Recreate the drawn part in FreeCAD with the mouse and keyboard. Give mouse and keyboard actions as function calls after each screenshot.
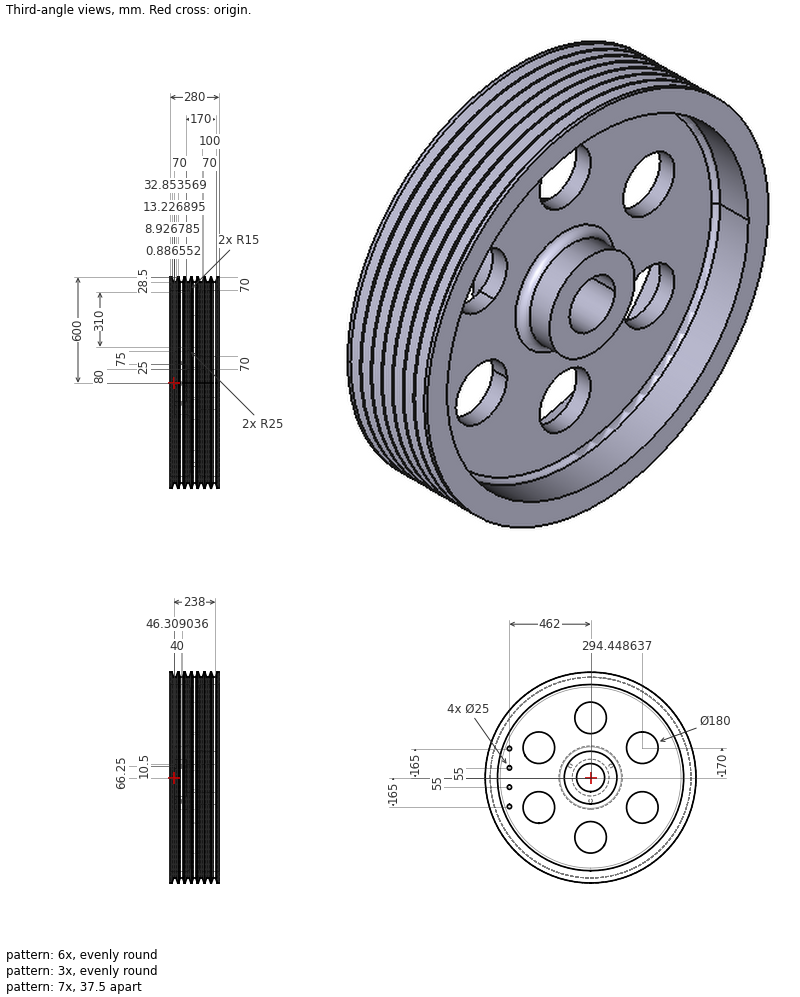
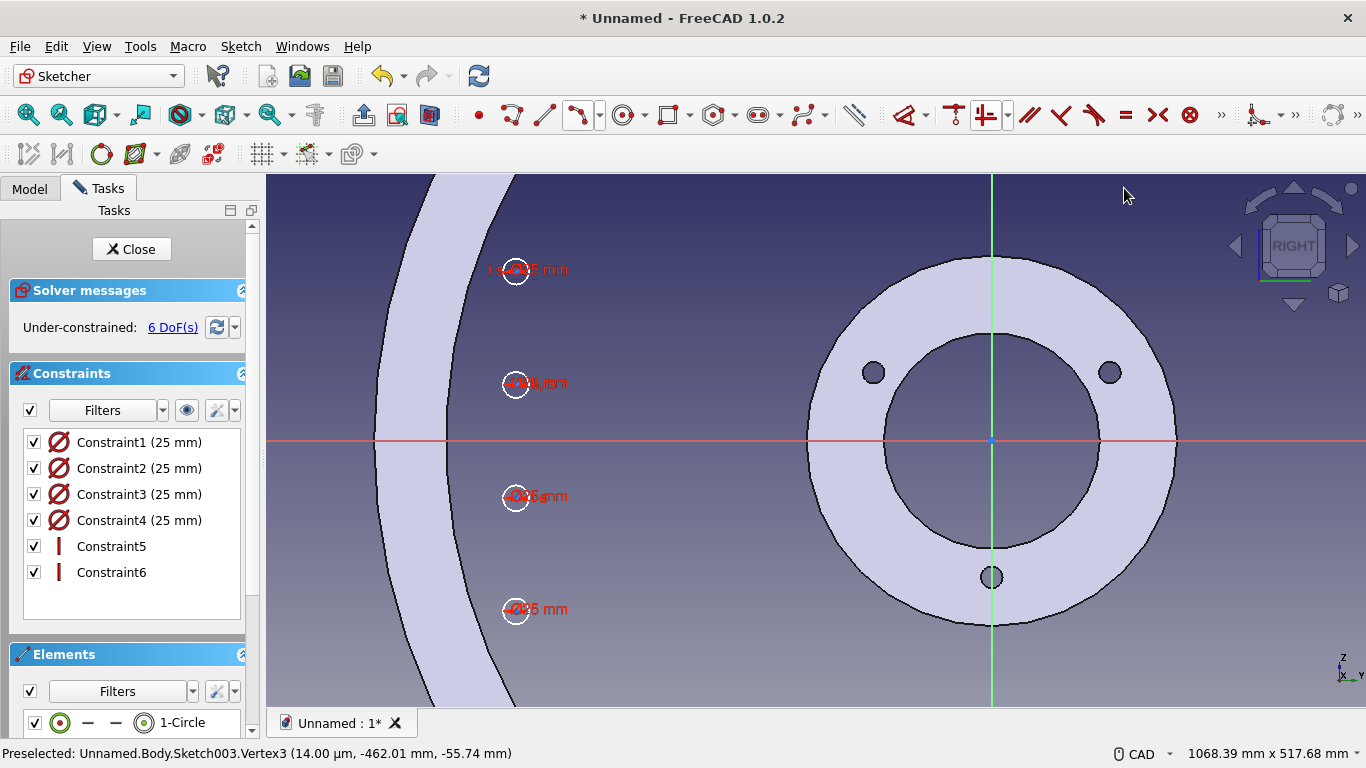
click(516, 498)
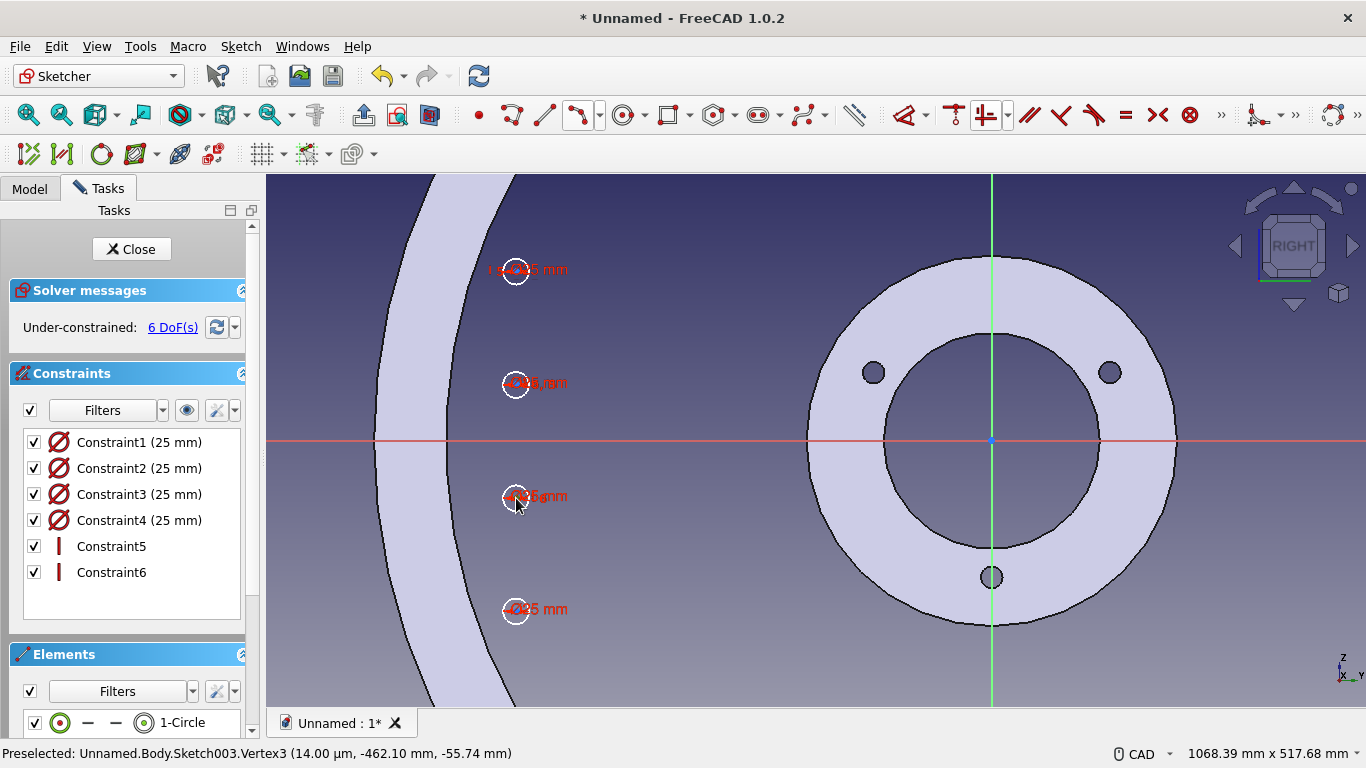
click(516, 611)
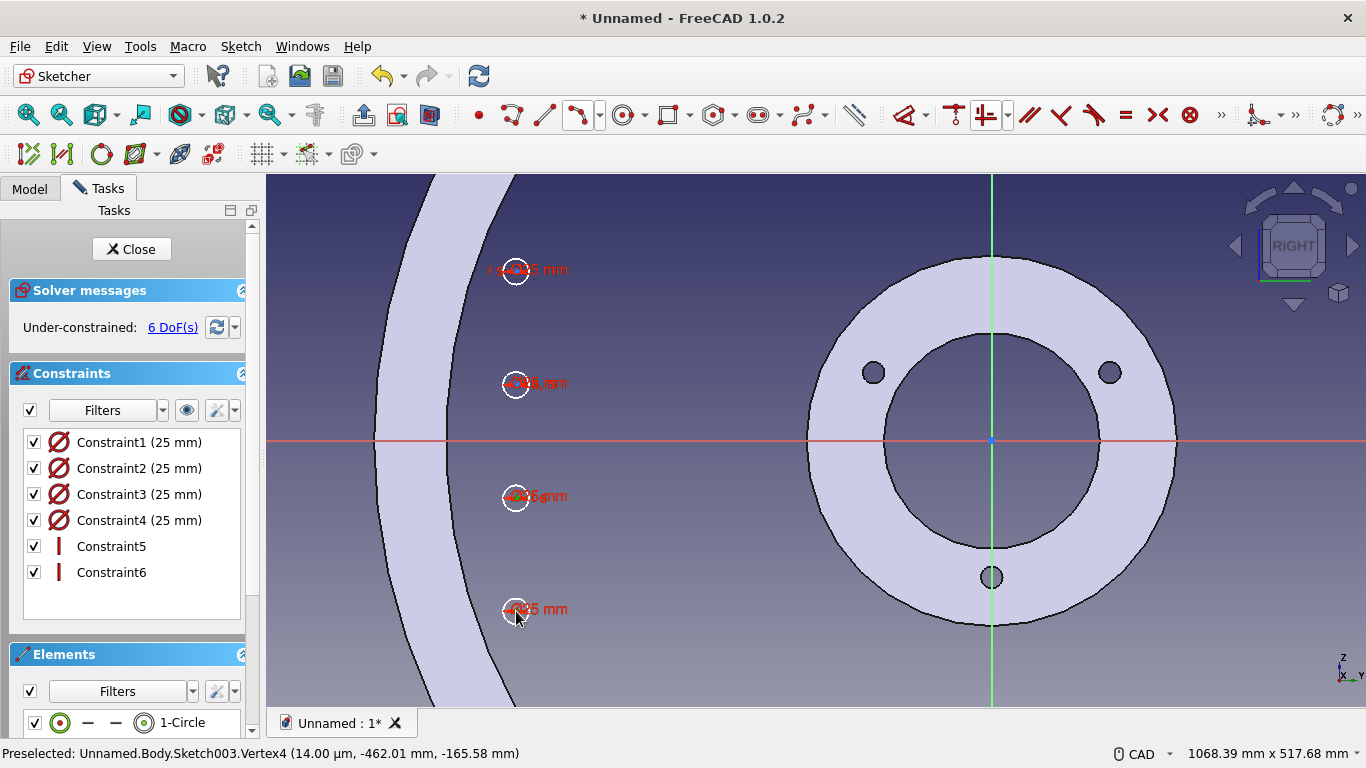
click(1008, 116)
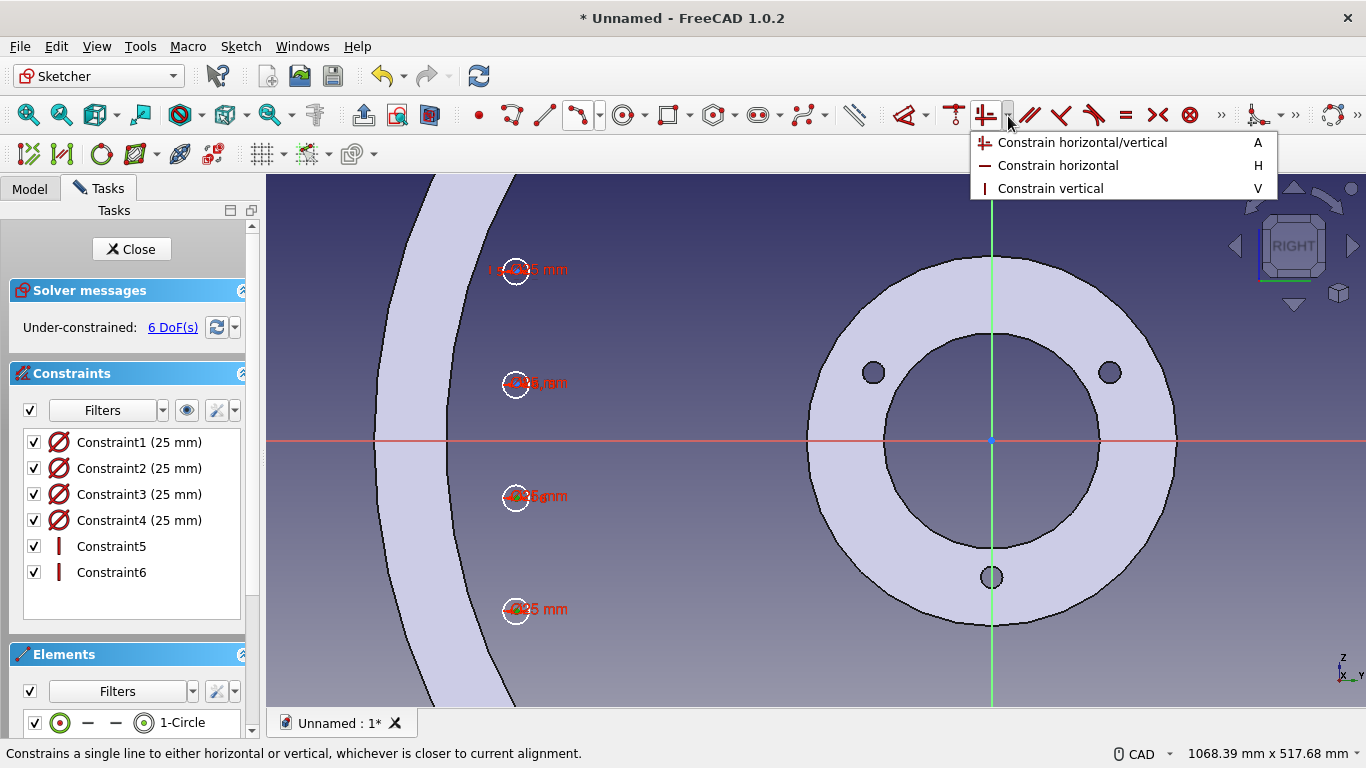
click(1124, 188)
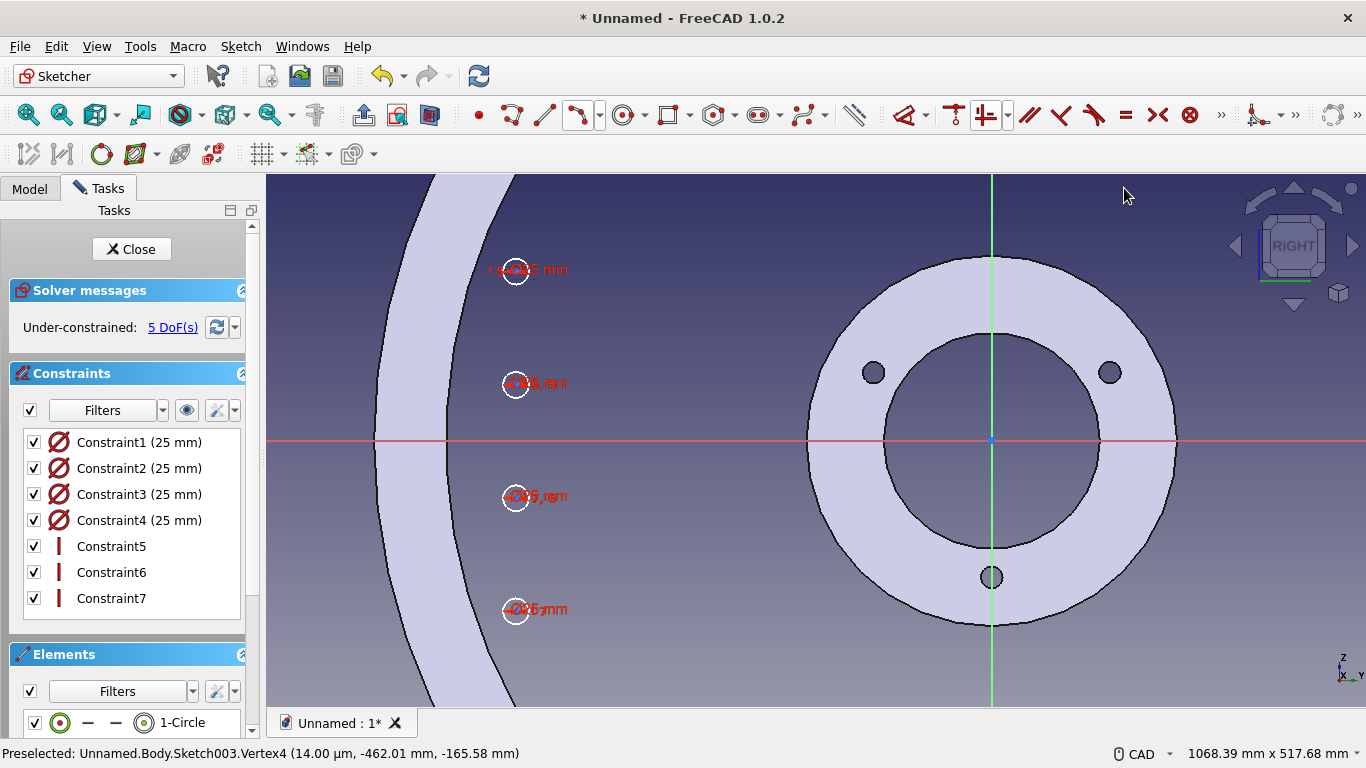
click(904, 116)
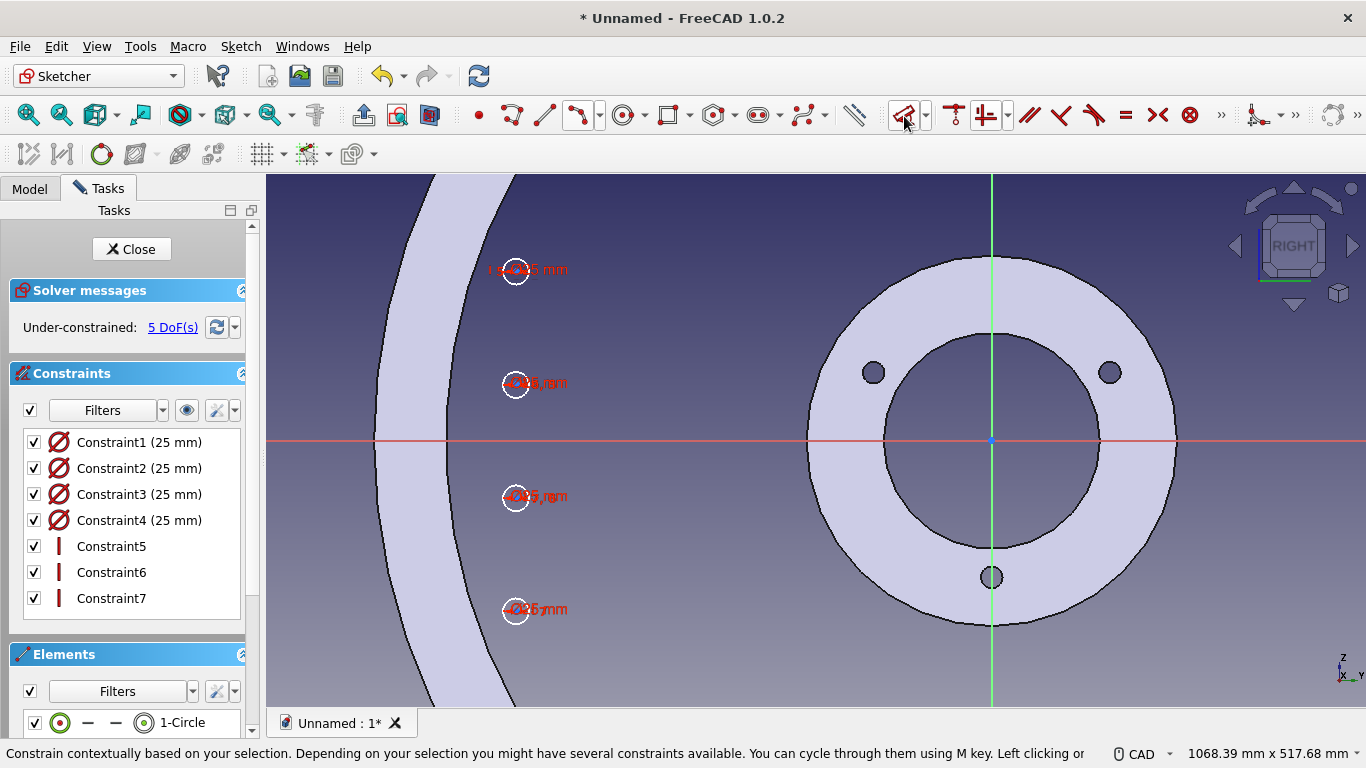
click(516, 385)
click(1026, 413)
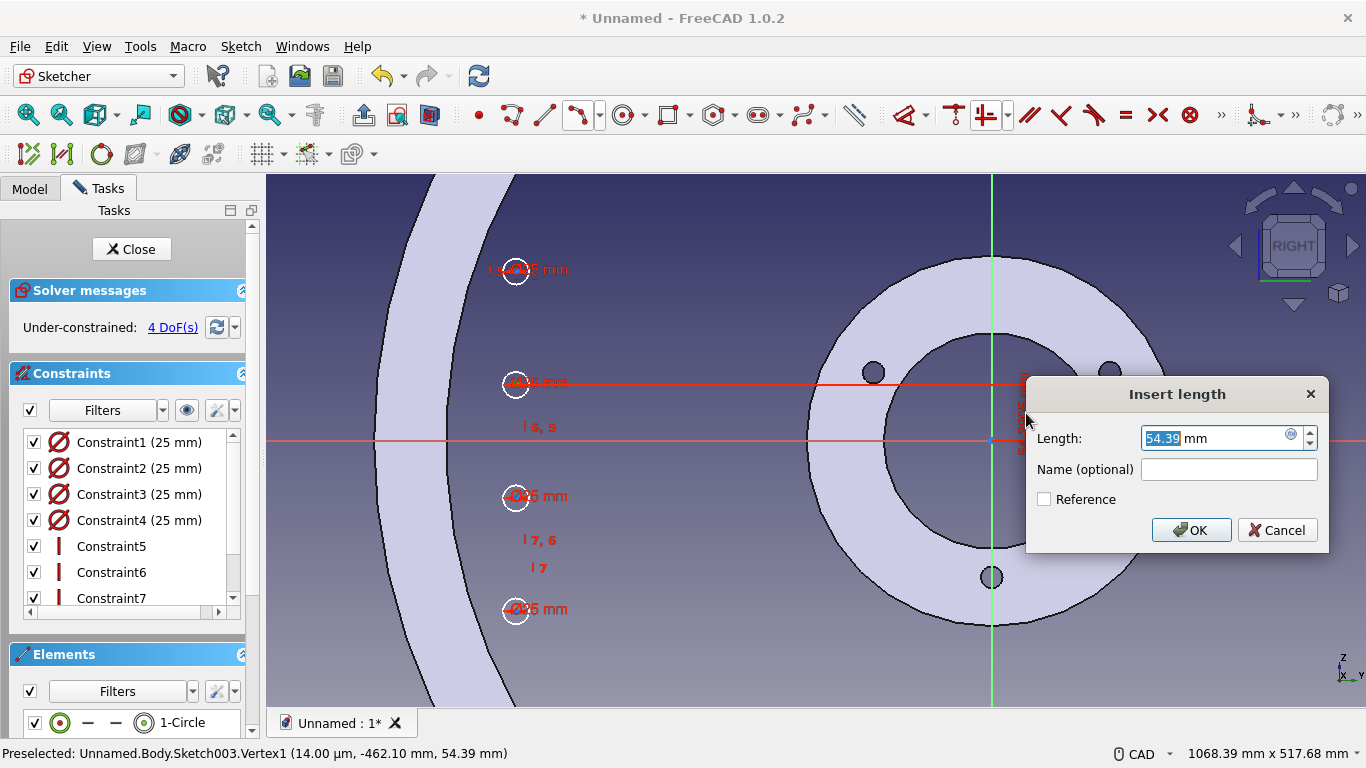
text(55)
key(Return)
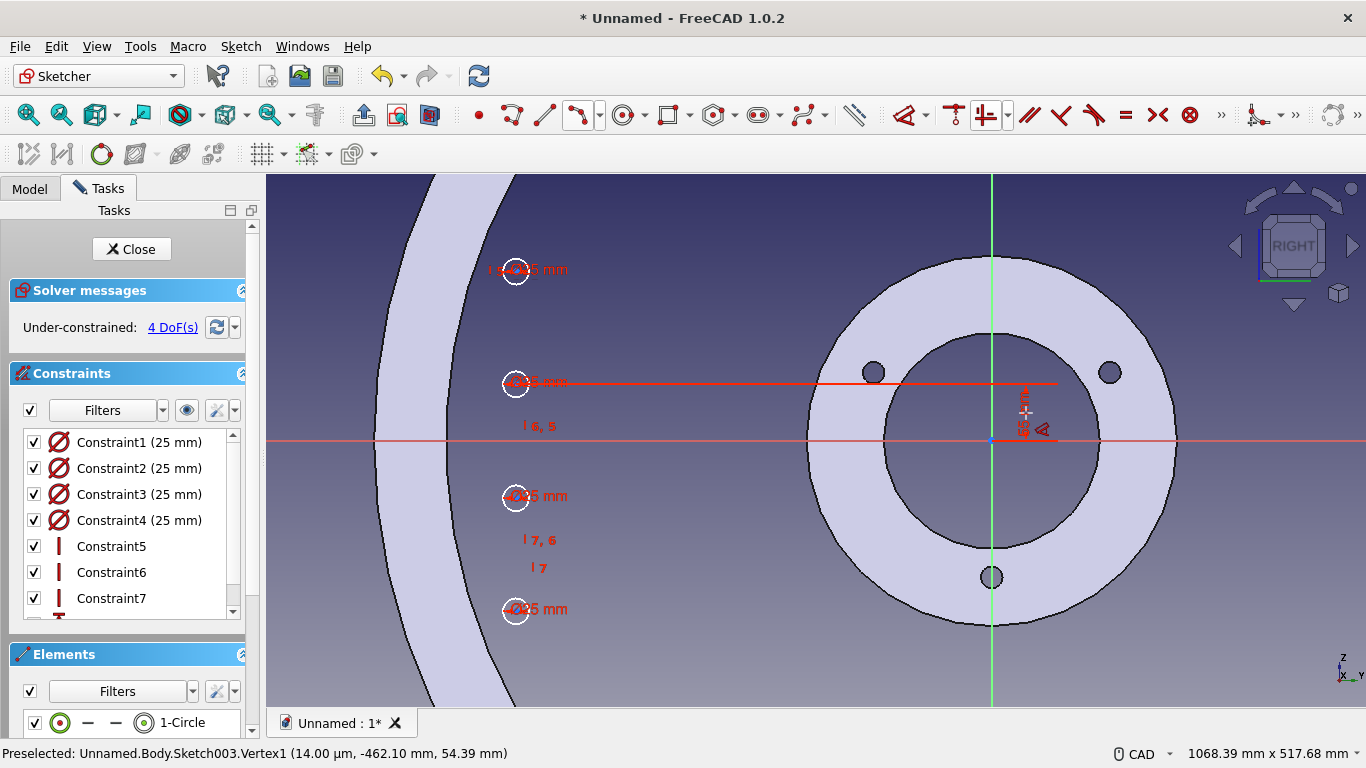
click(516, 498)
click(1026, 470)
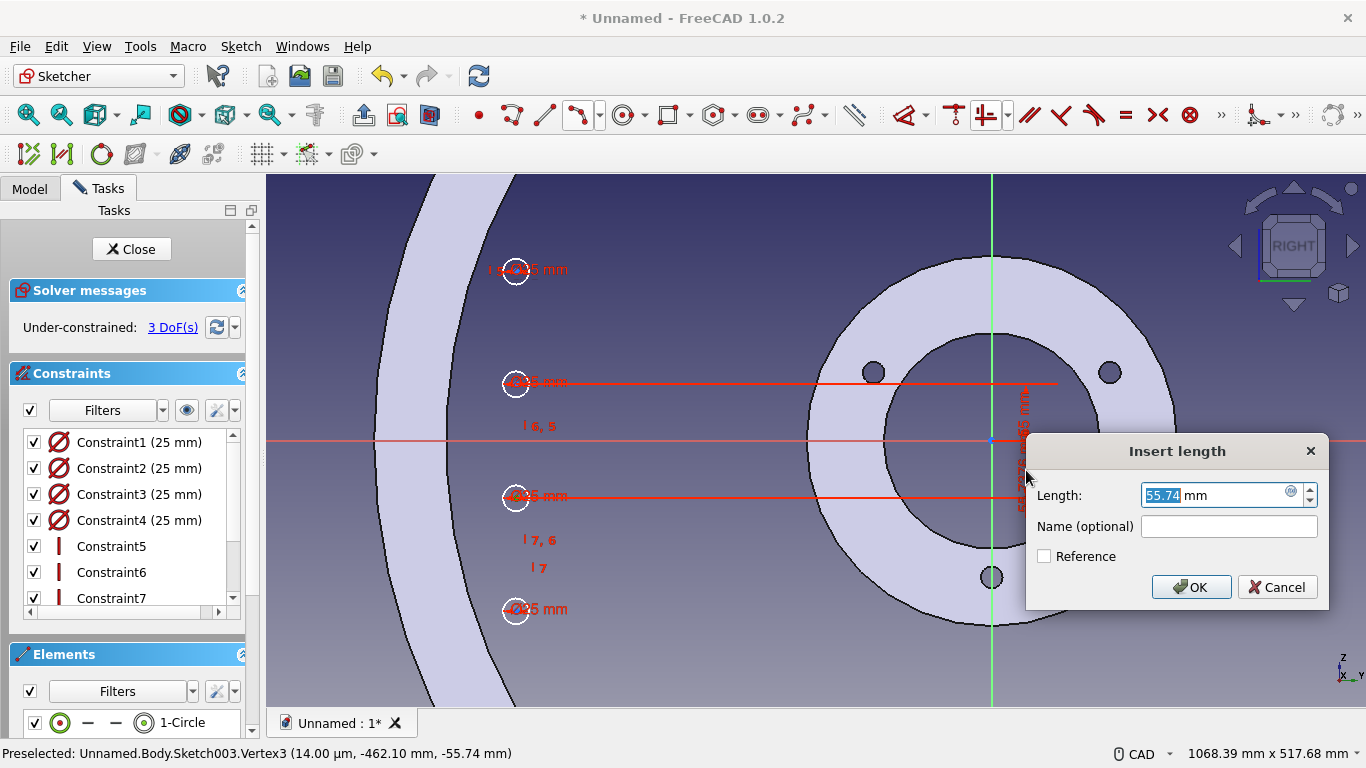
text(55)
key(Return)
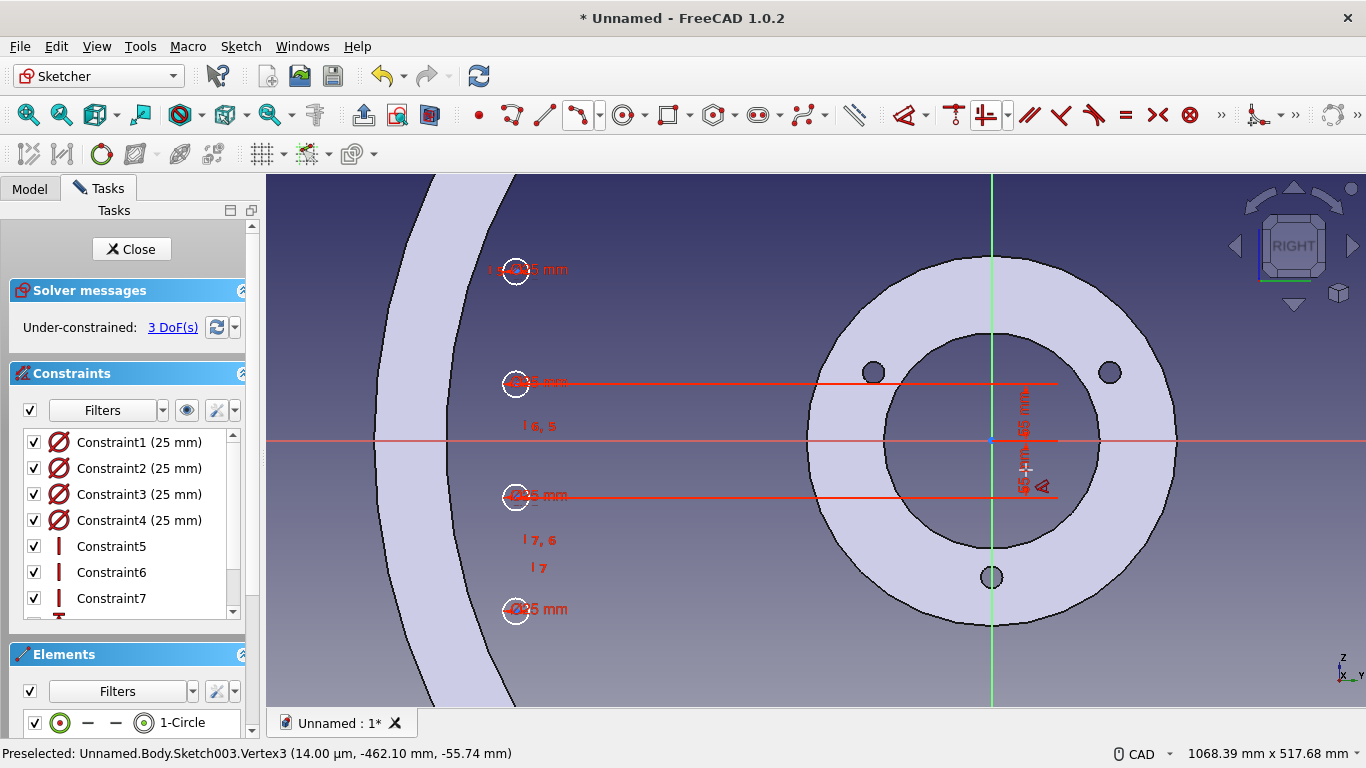
click(516, 384)
click(754, 350)